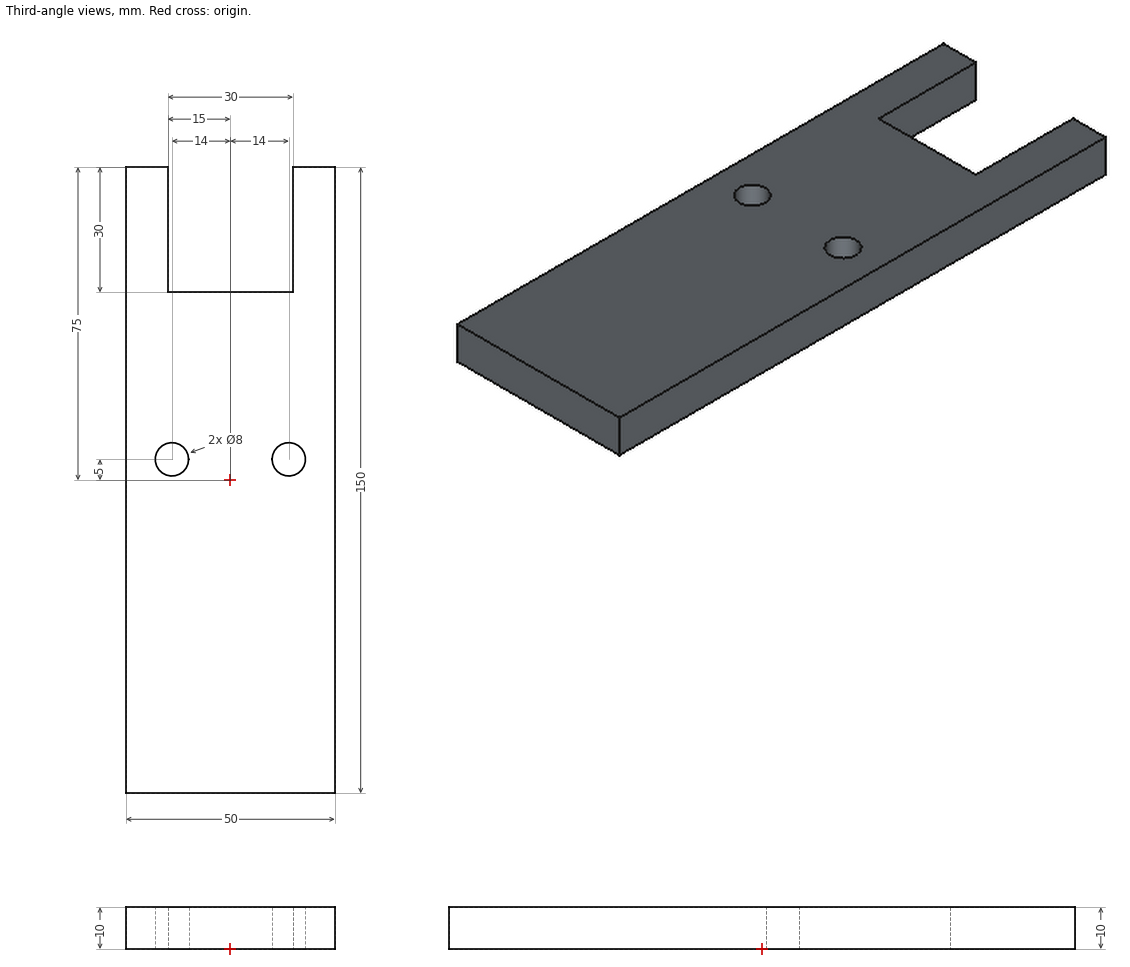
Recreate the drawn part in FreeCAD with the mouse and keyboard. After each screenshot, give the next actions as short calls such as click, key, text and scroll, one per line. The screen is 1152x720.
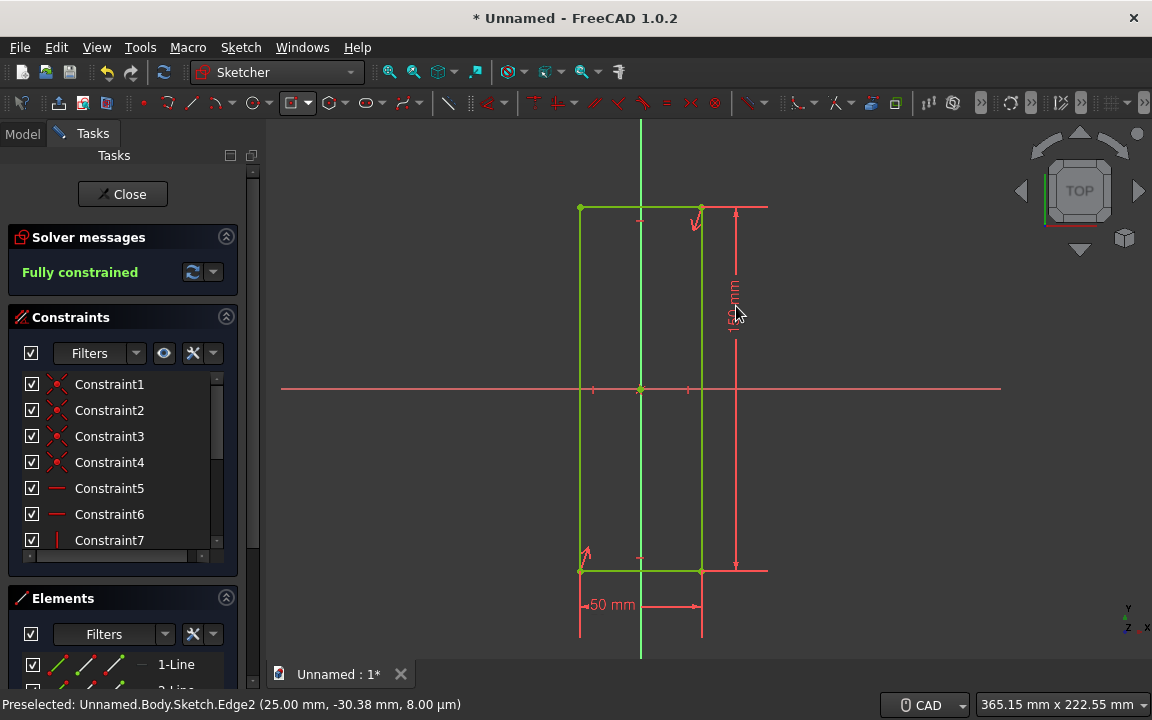
click(123, 194)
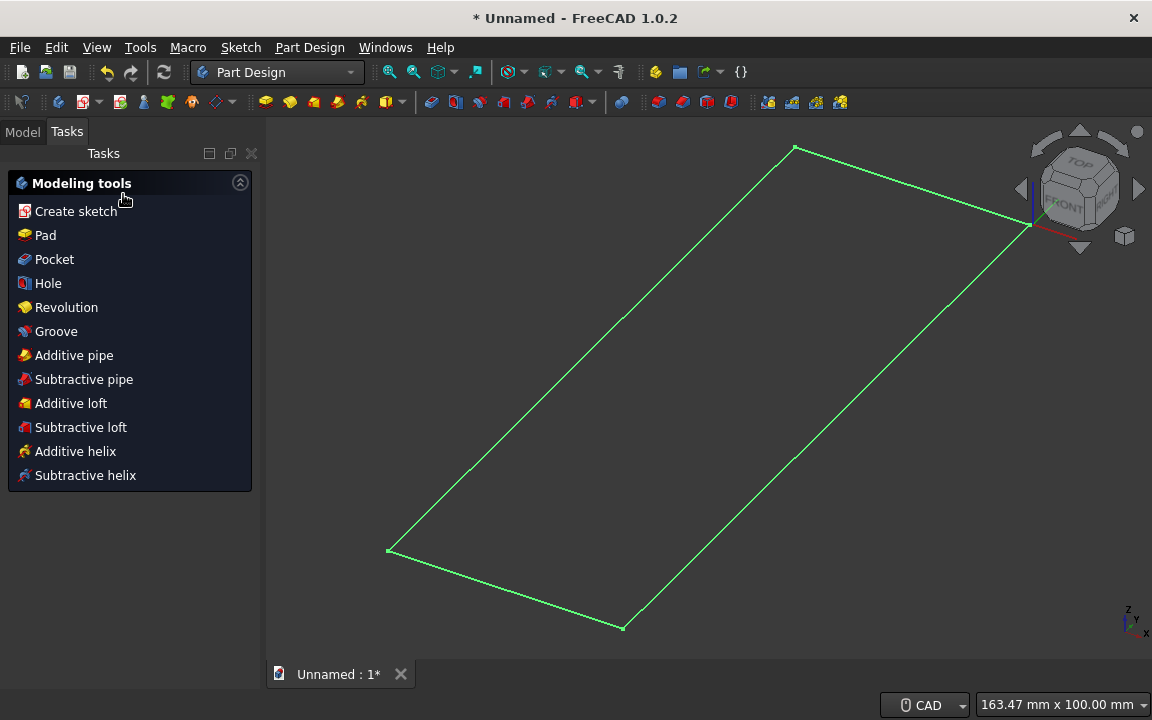
click(266, 102)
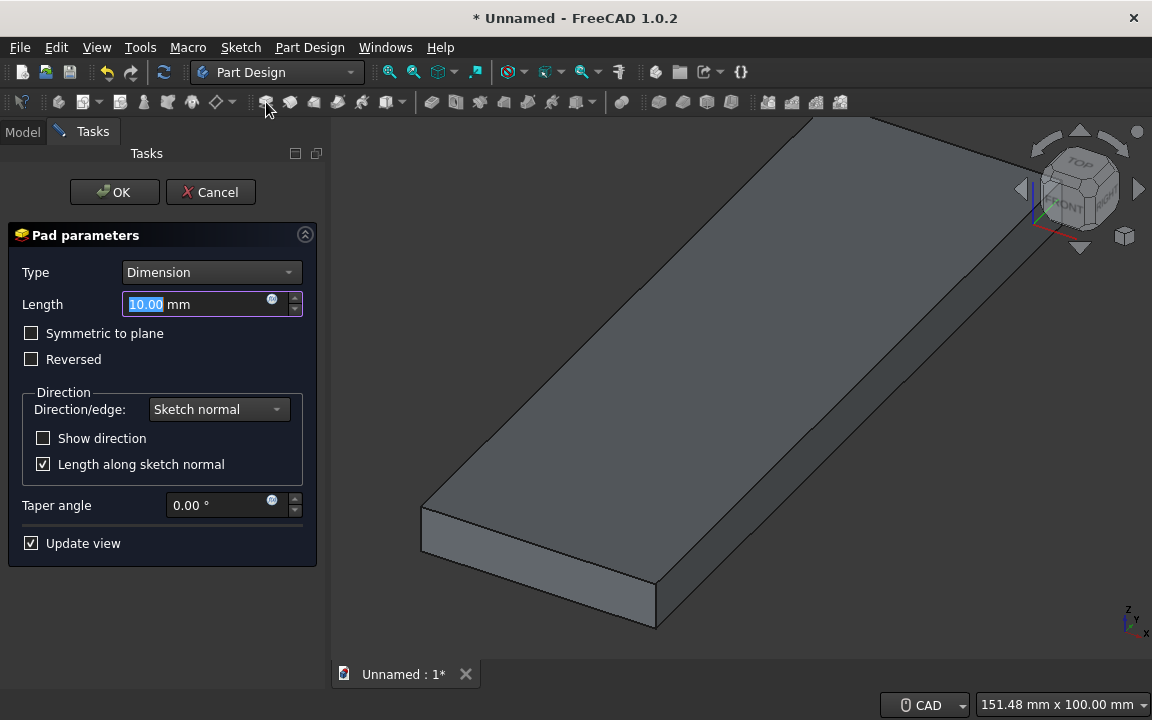
text(10)
key(Tab)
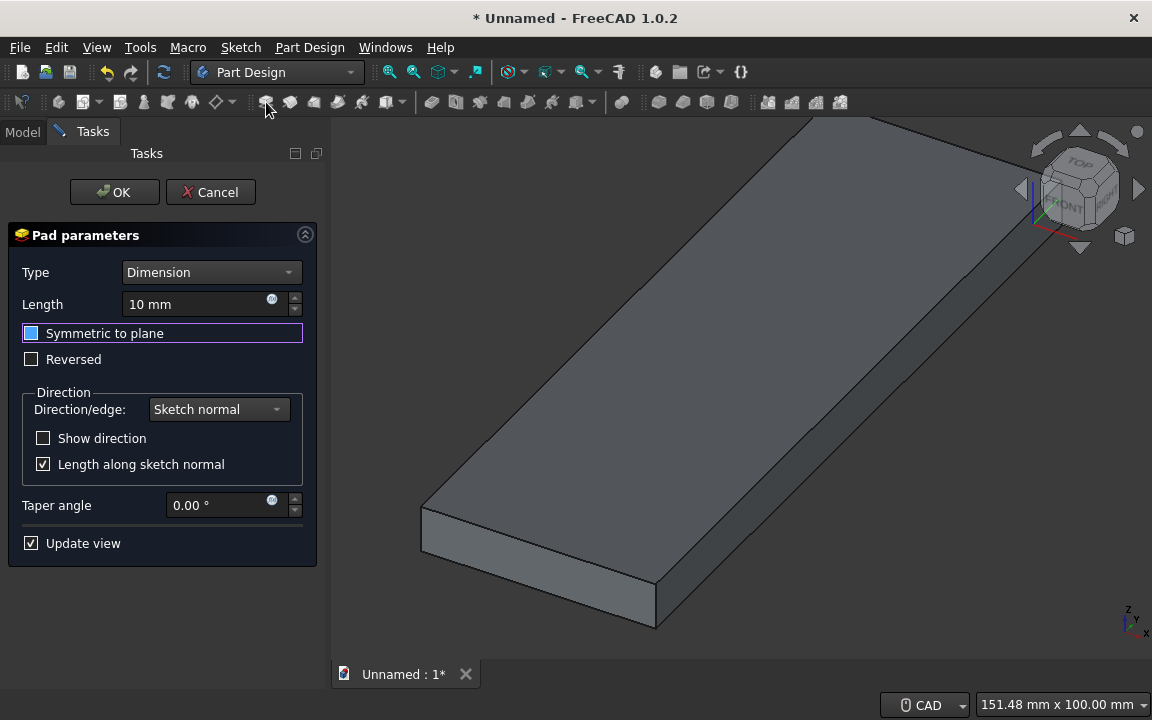
click(115, 192)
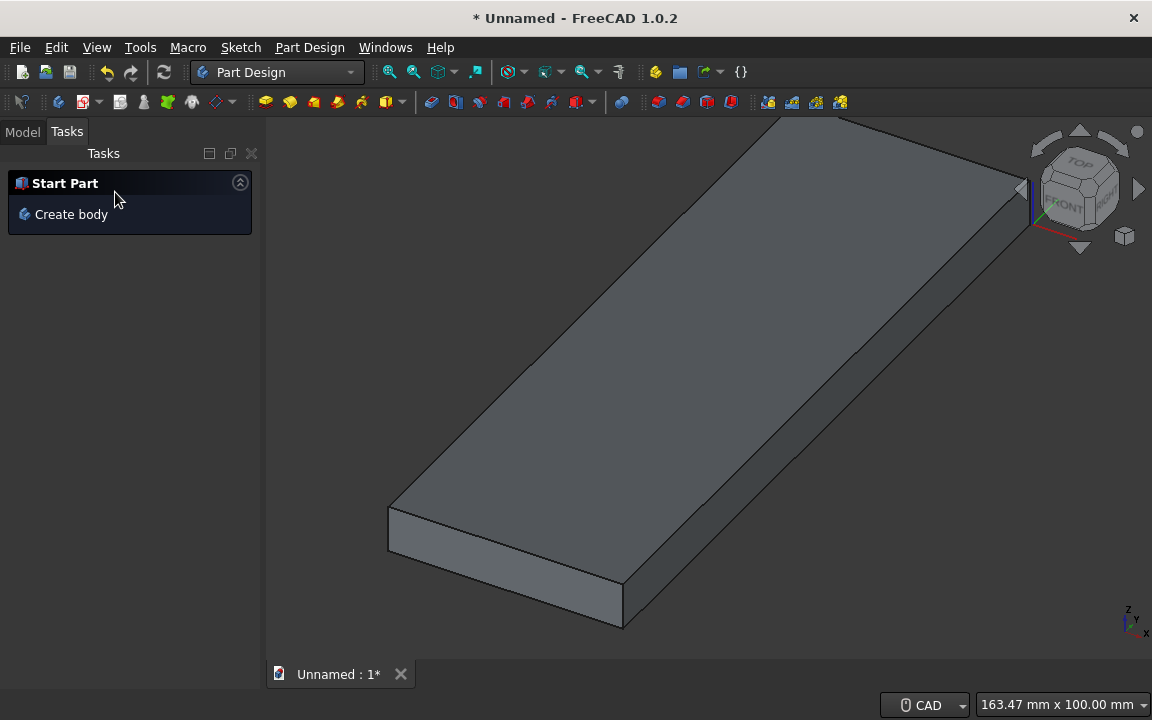
key(v)
key(f)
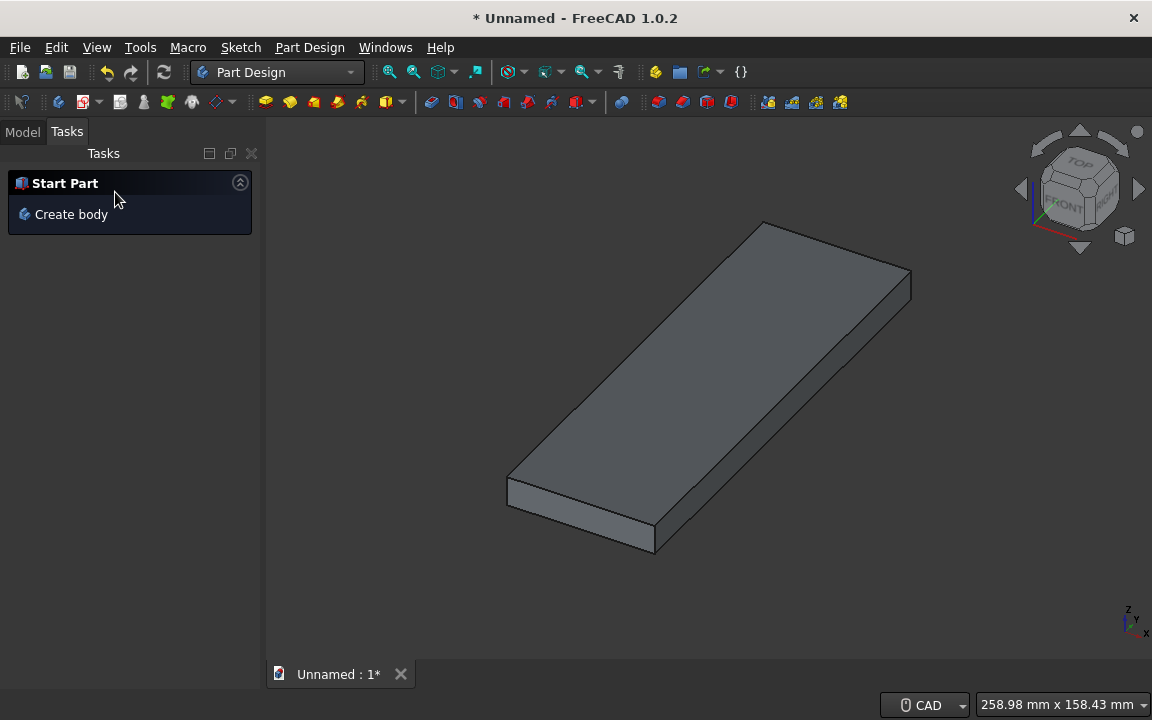
click(782, 300)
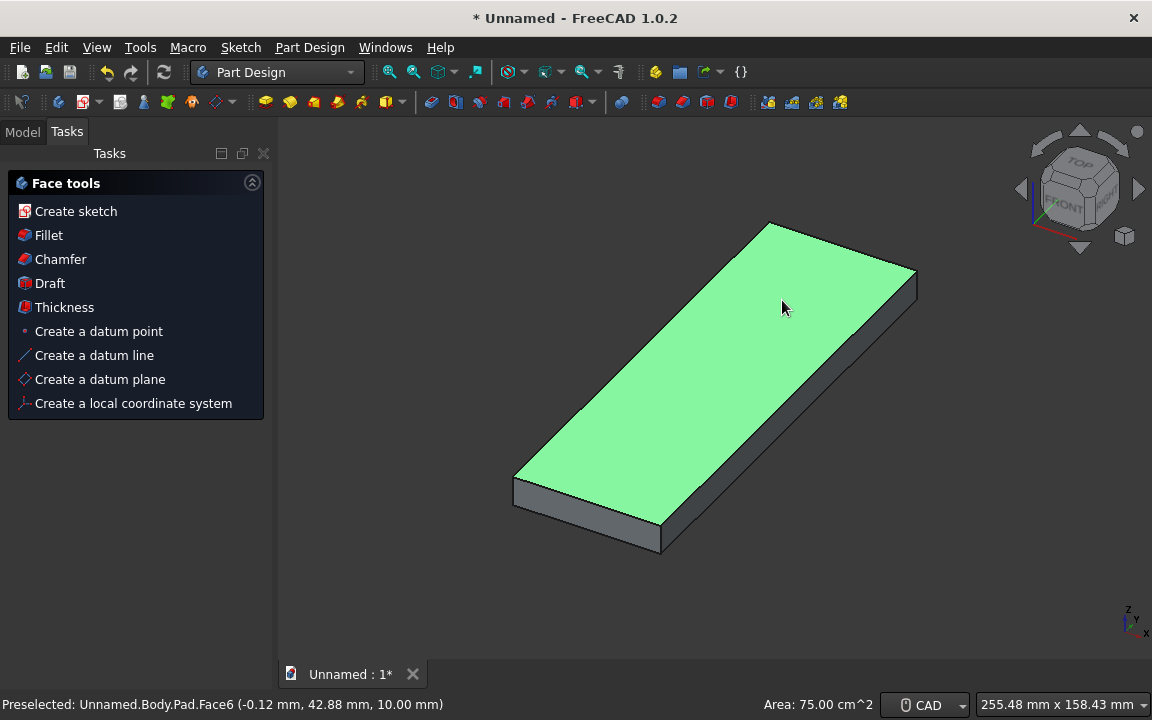
click(84, 102)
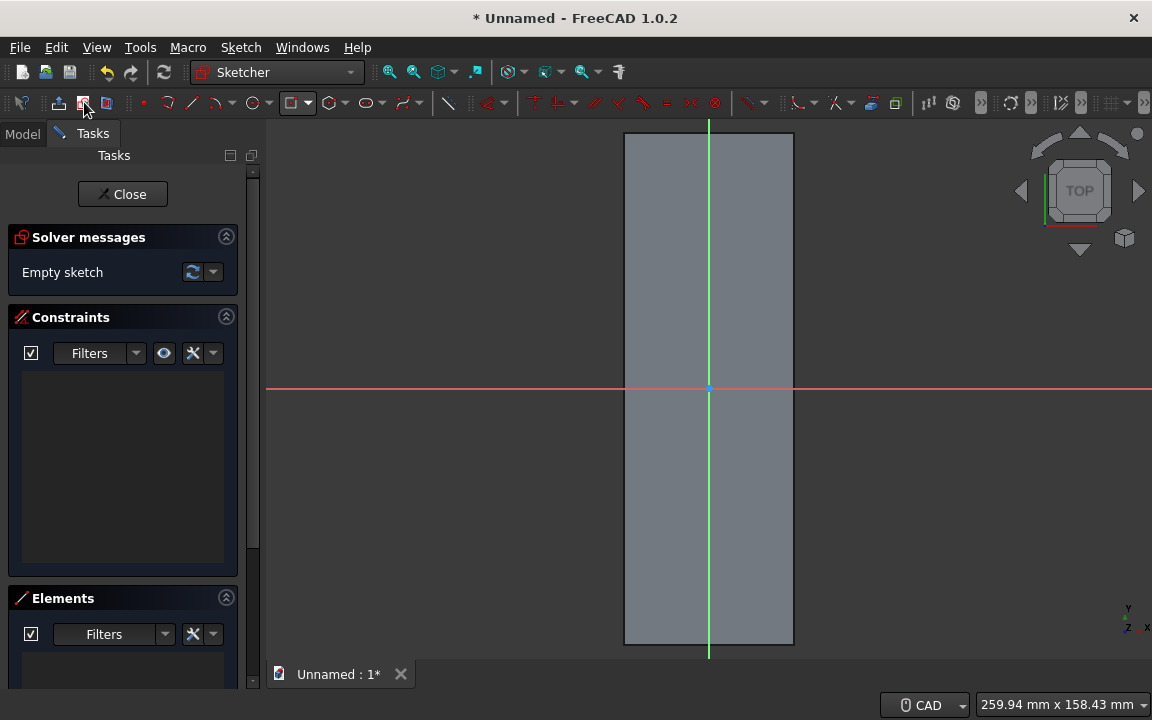
scroll(640, 389, down, 5)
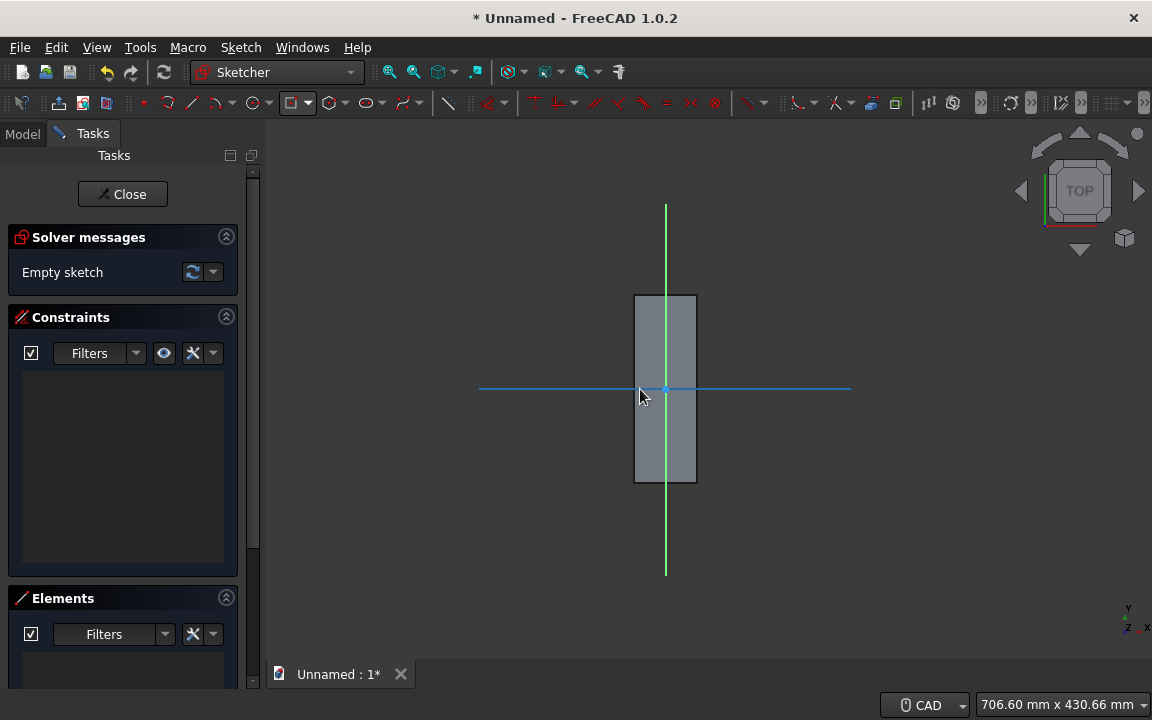
scroll(669, 305, up, 11)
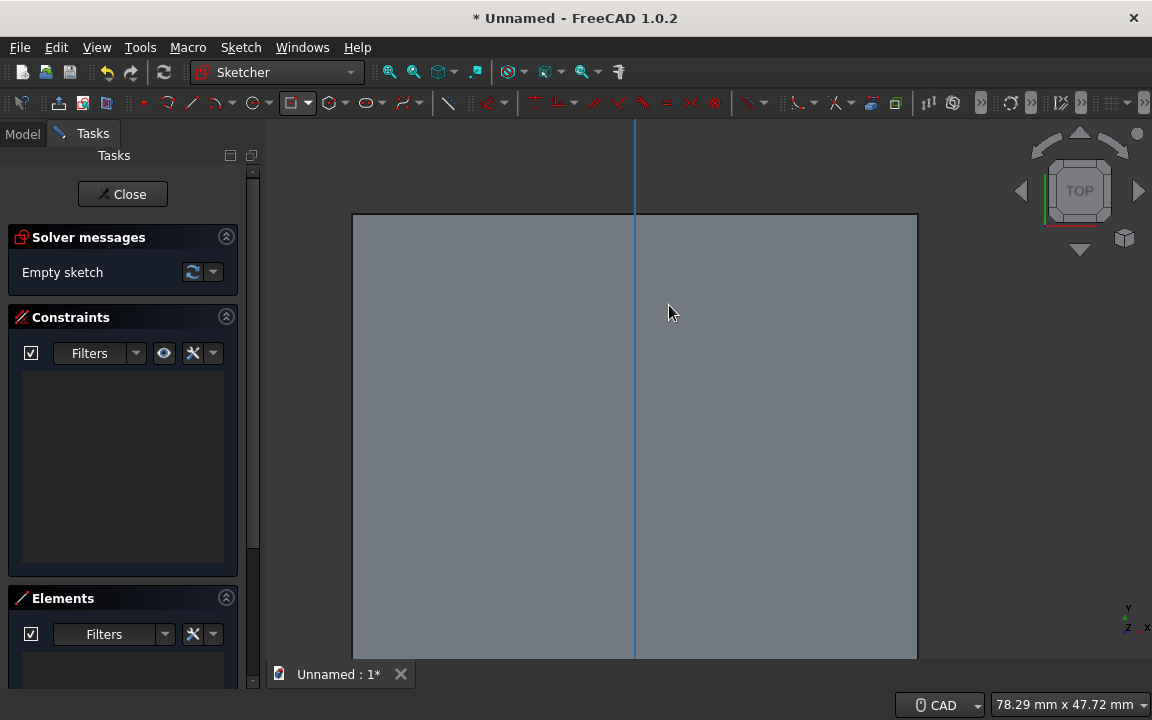
key(g)
key(r)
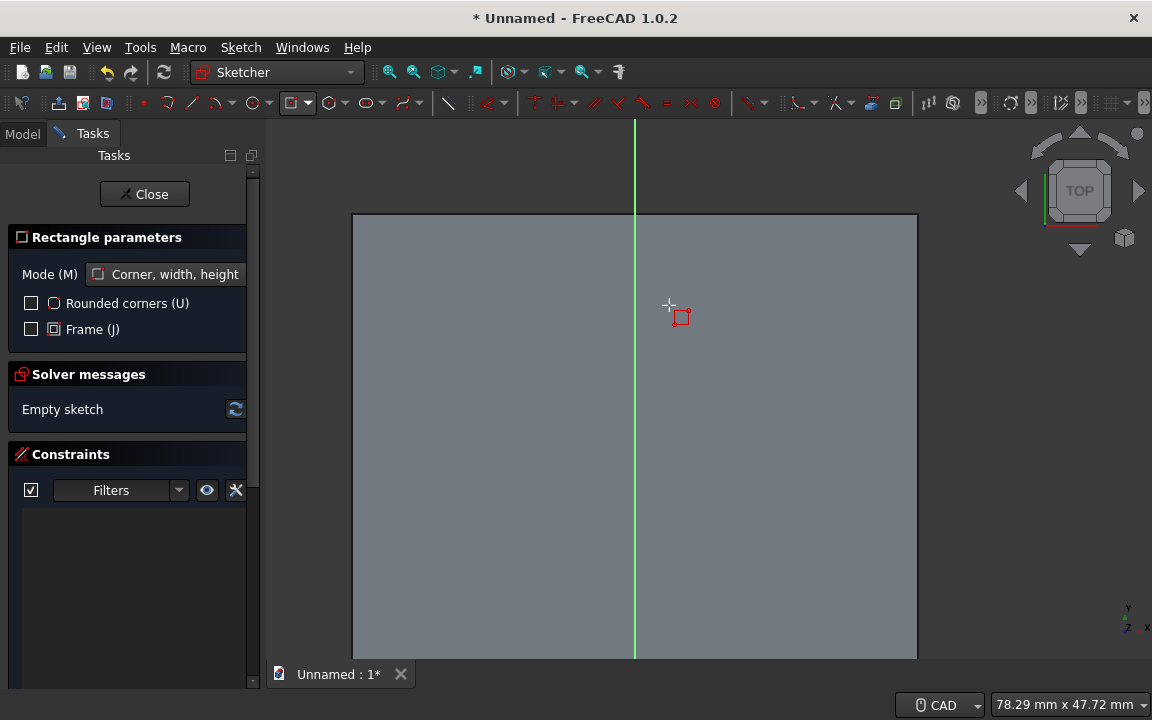
click(465, 214)
click(805, 554)
key(Escape)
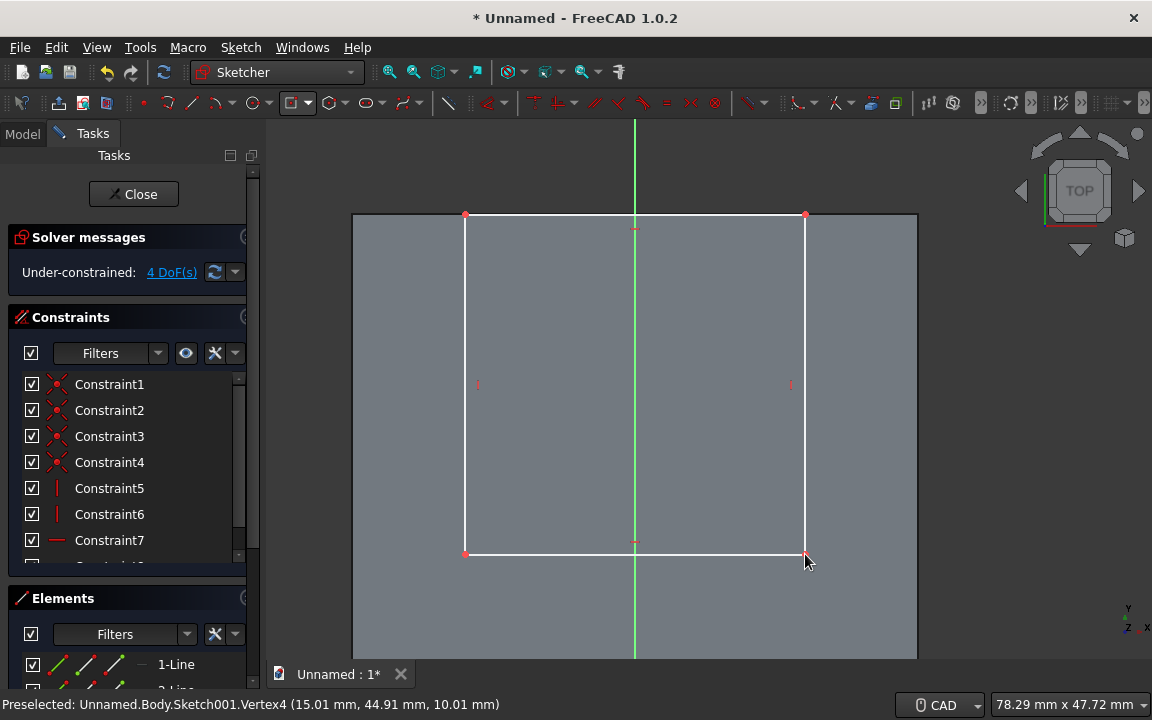
key(d)